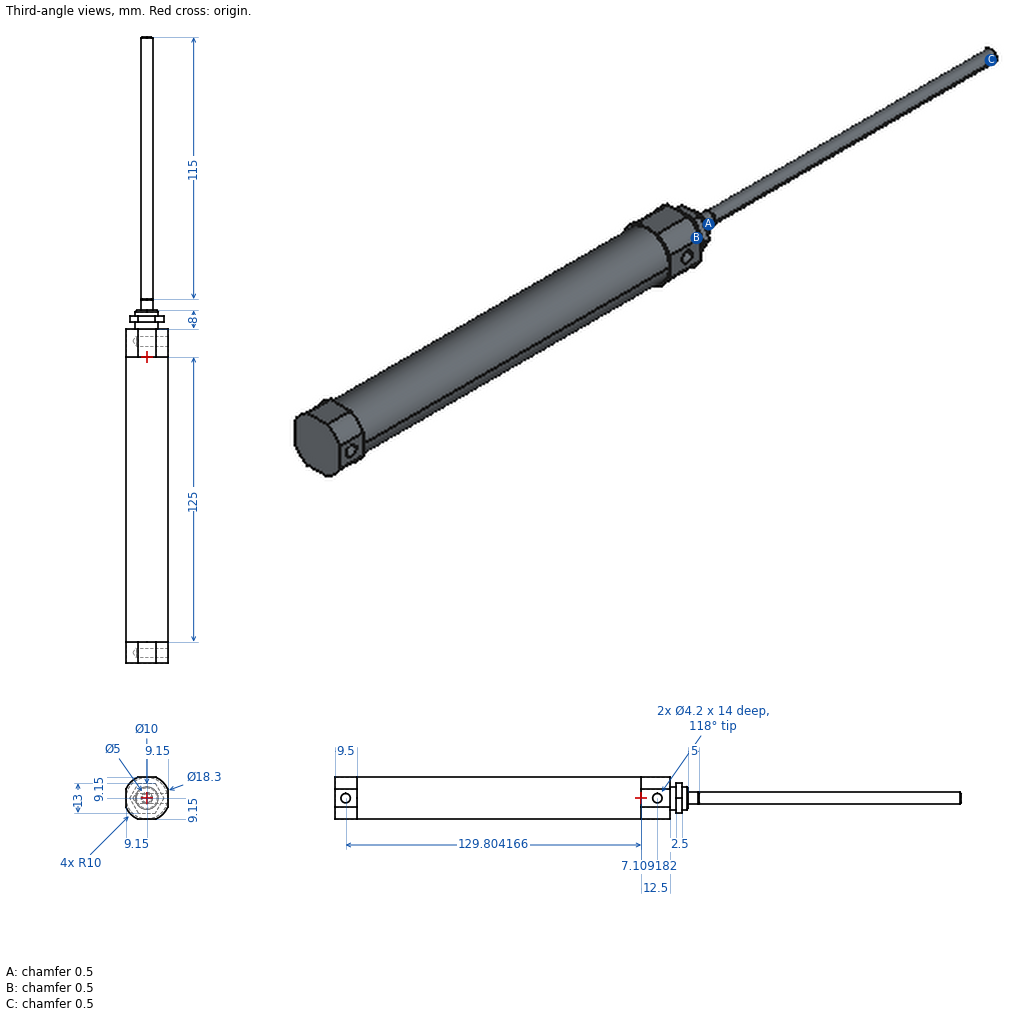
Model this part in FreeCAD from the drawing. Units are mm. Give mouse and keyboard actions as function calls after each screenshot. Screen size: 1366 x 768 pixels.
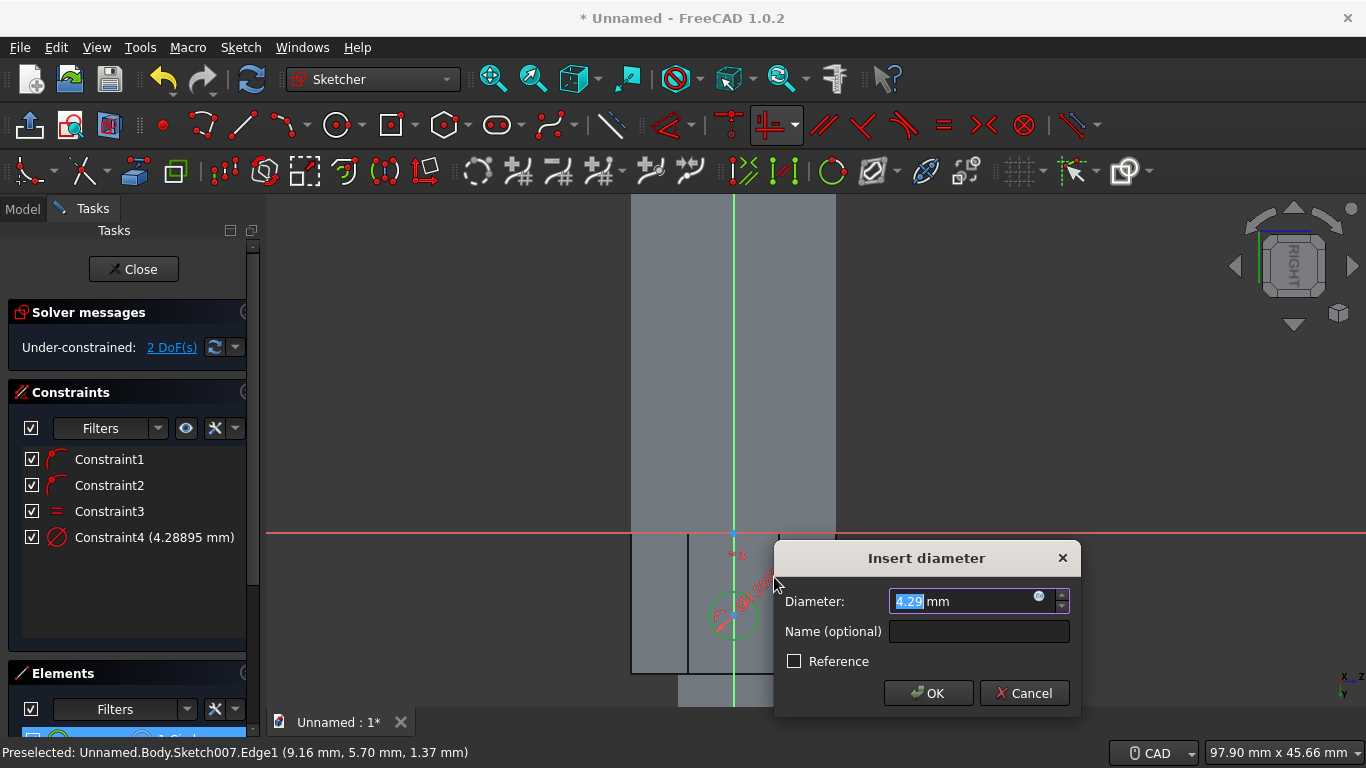
text(4.2)
key(Return)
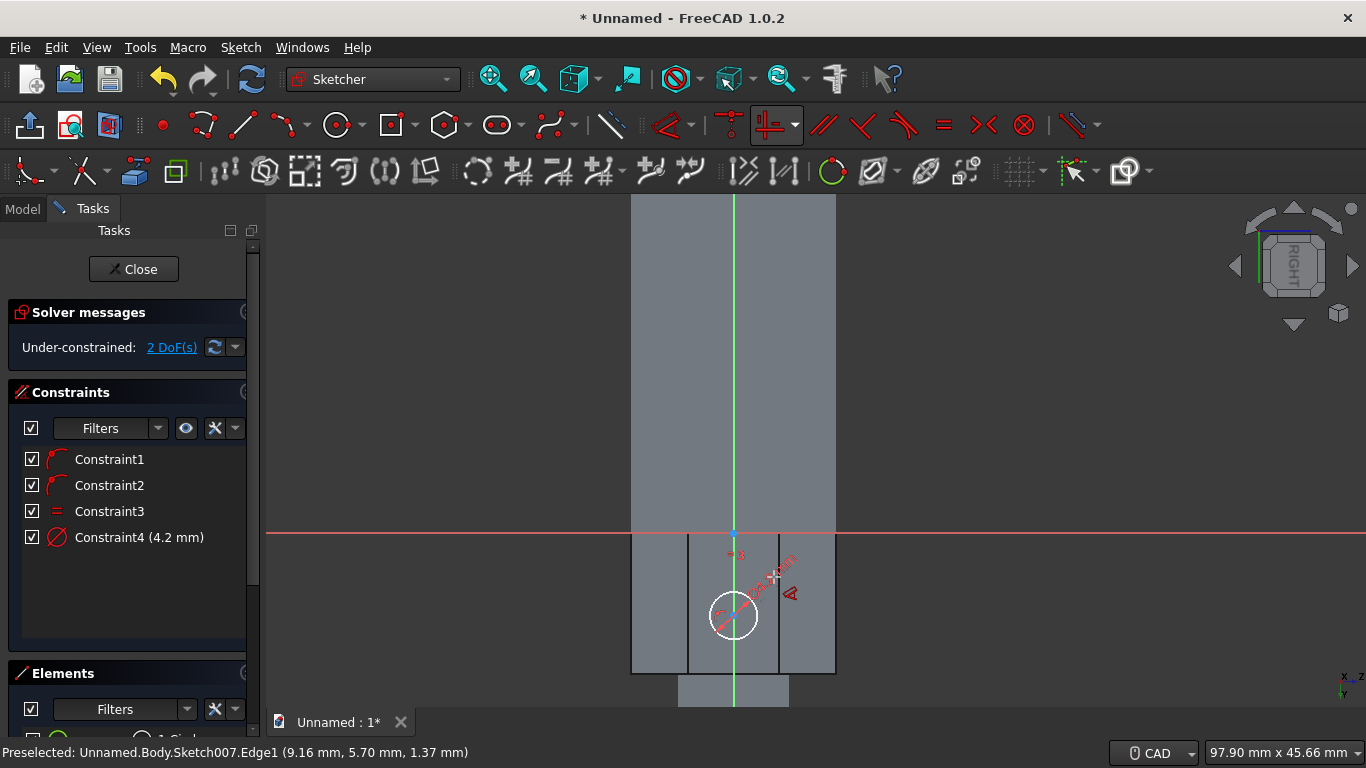
click(734, 616)
click(768, 555)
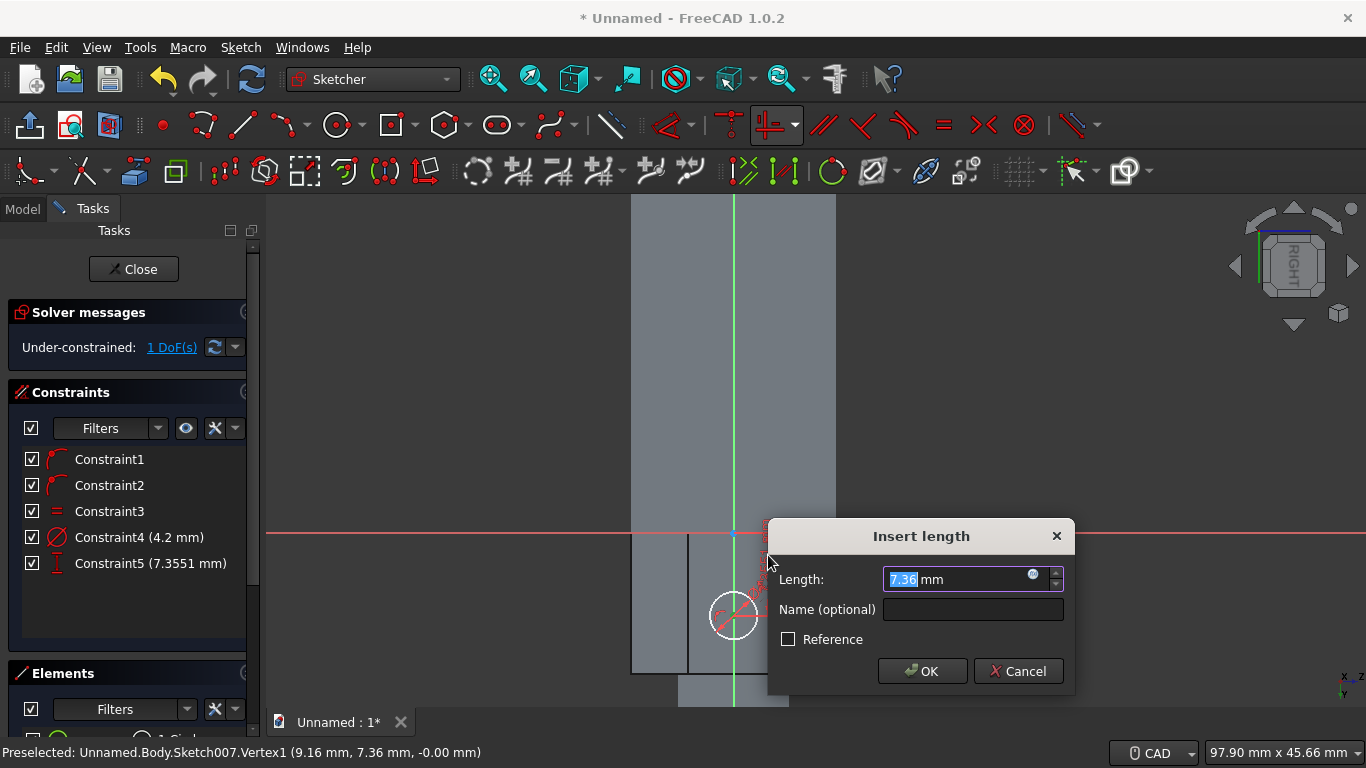
text(7.109182)
key(Return)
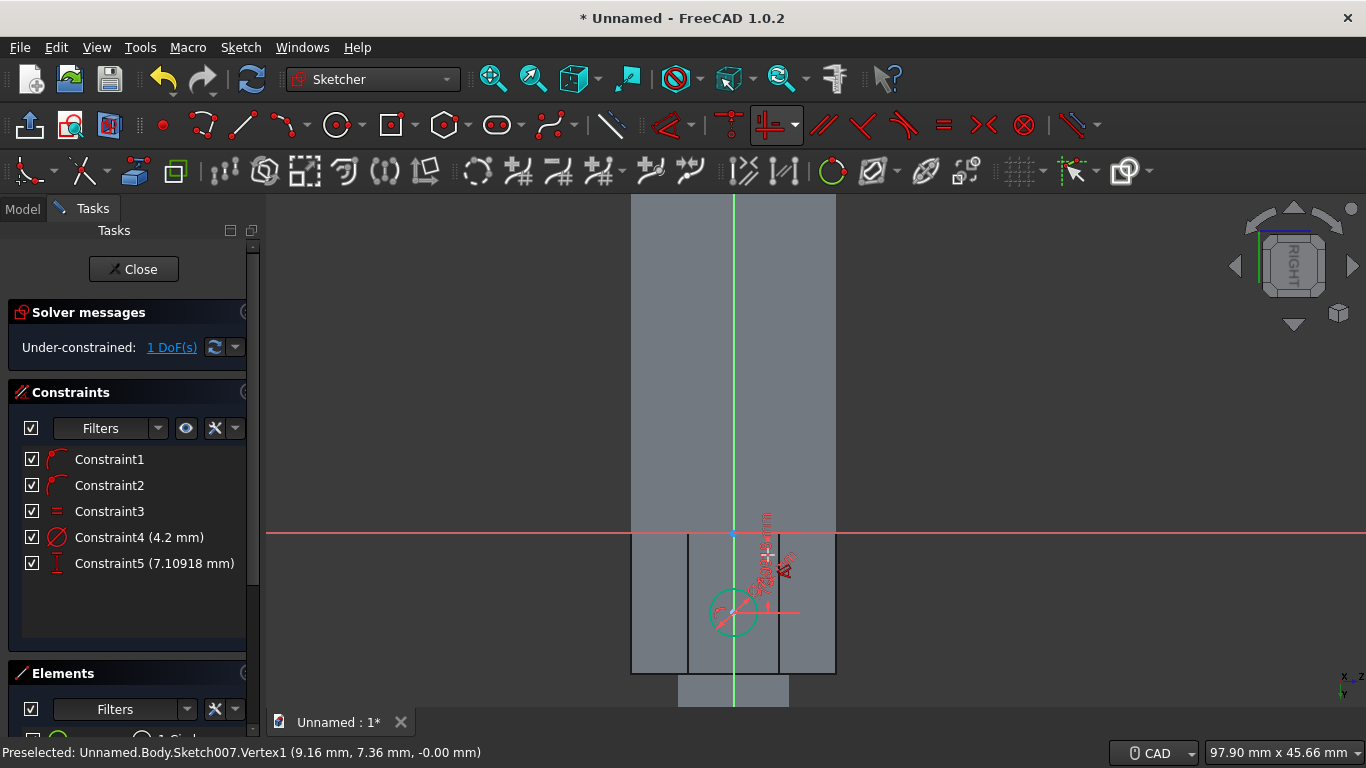
scroll(751, 604, down, 8)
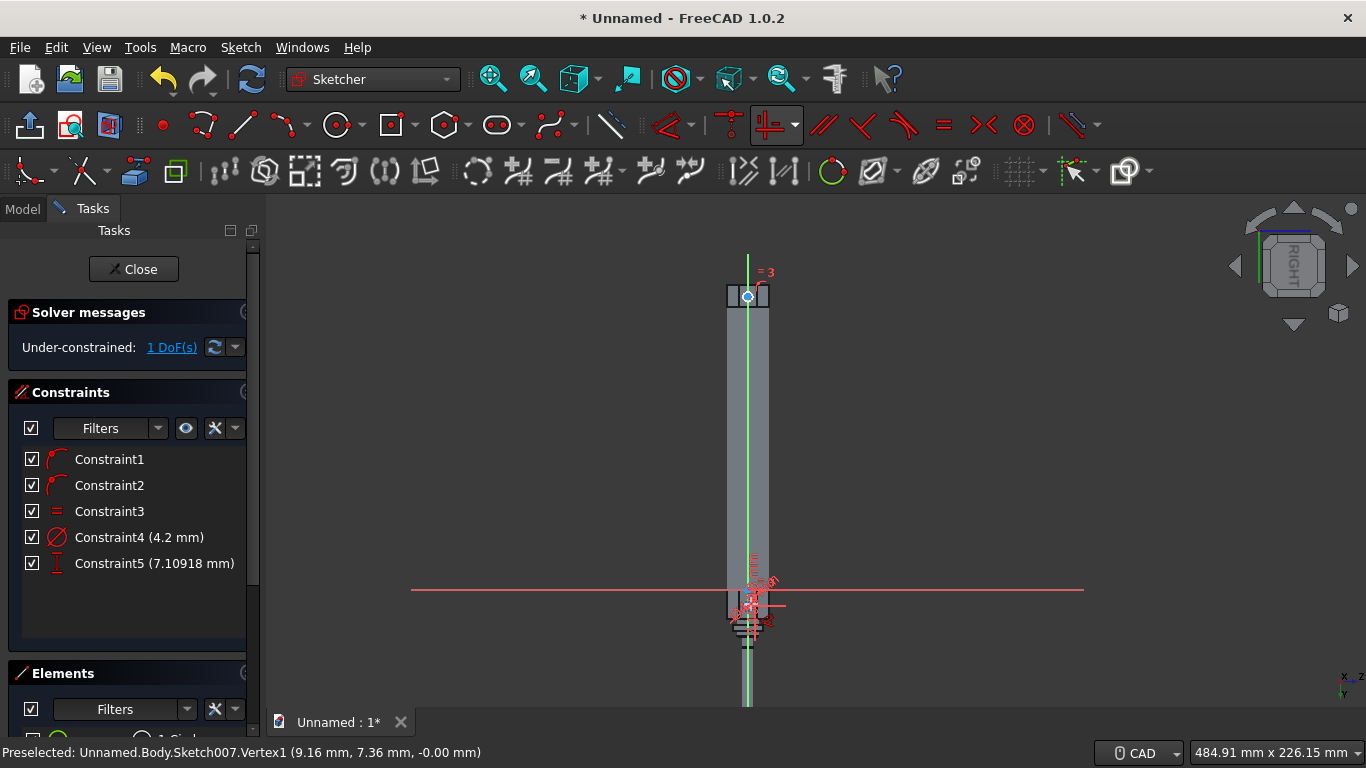
click(748, 297)
click(782, 444)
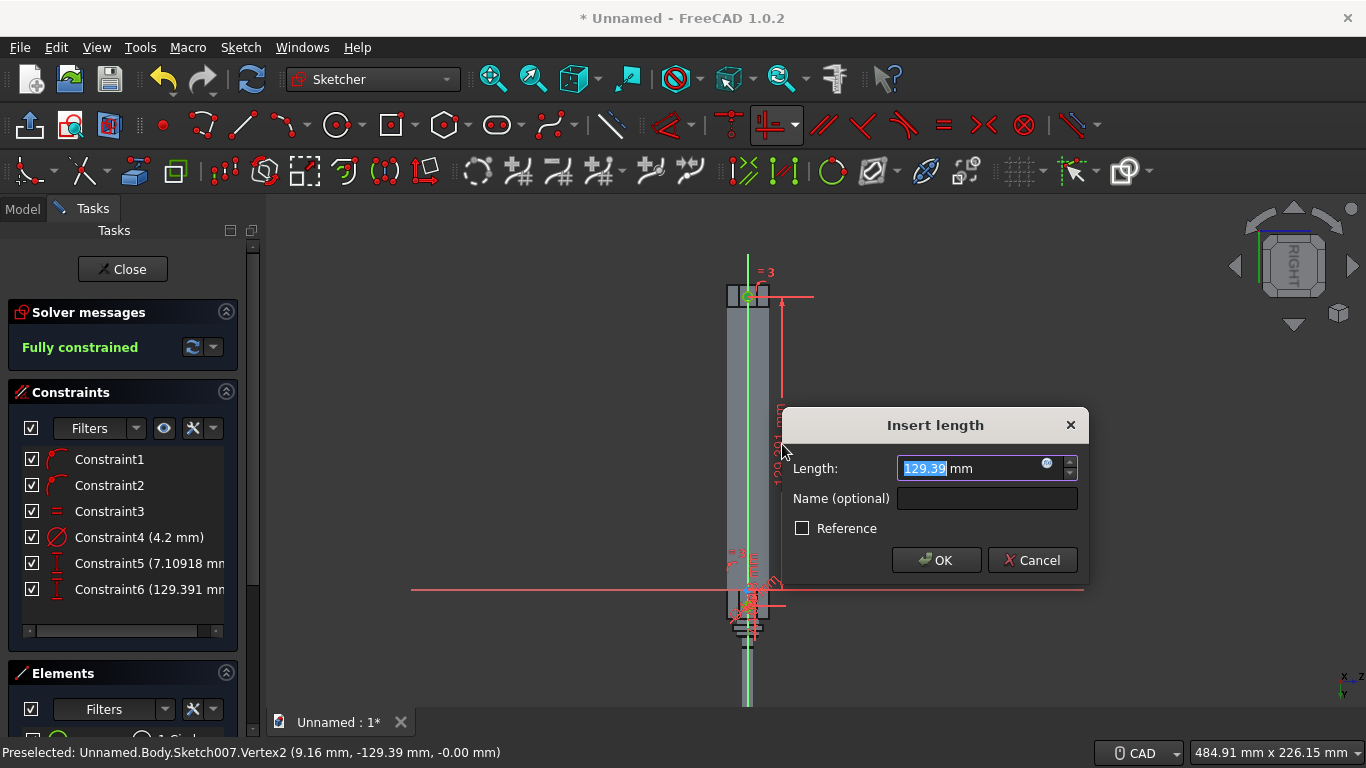
text(129.804166)
key(Return)
key(Escape)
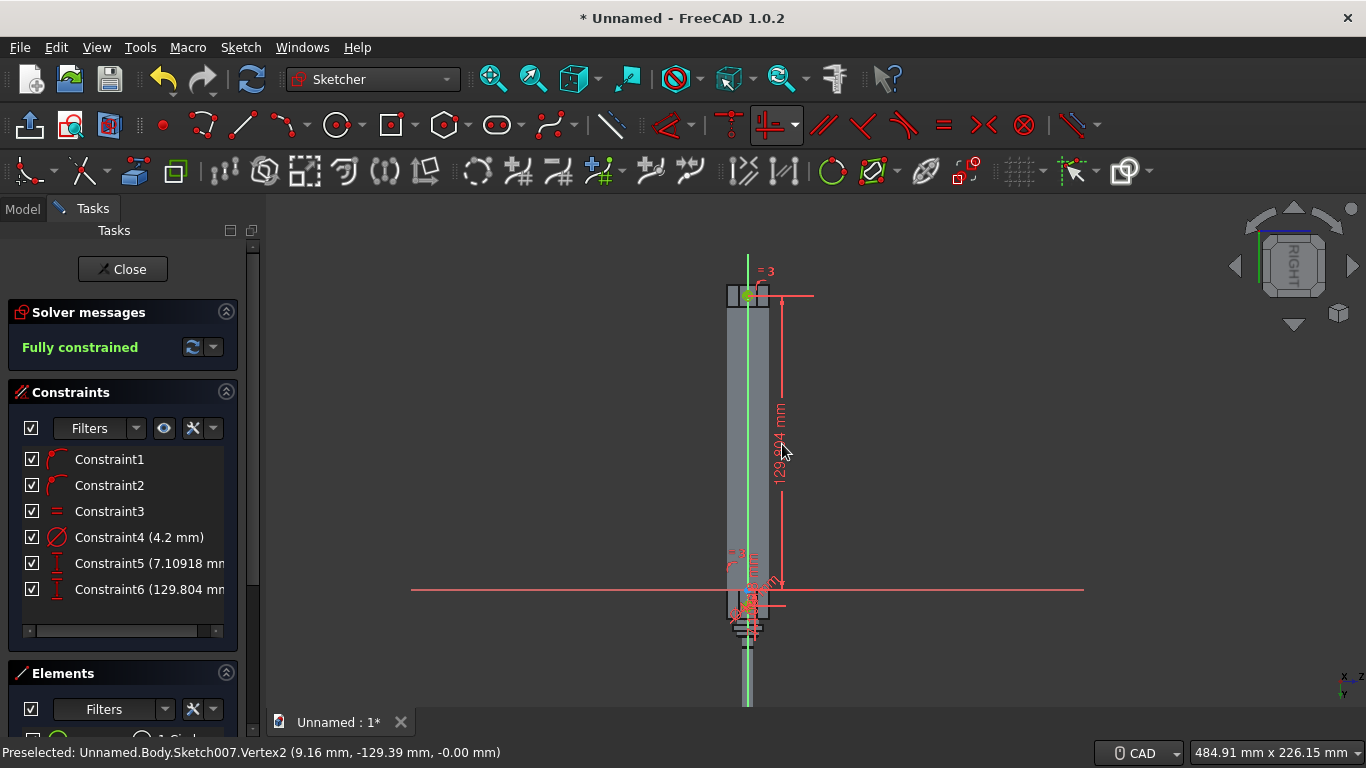
click(123, 269)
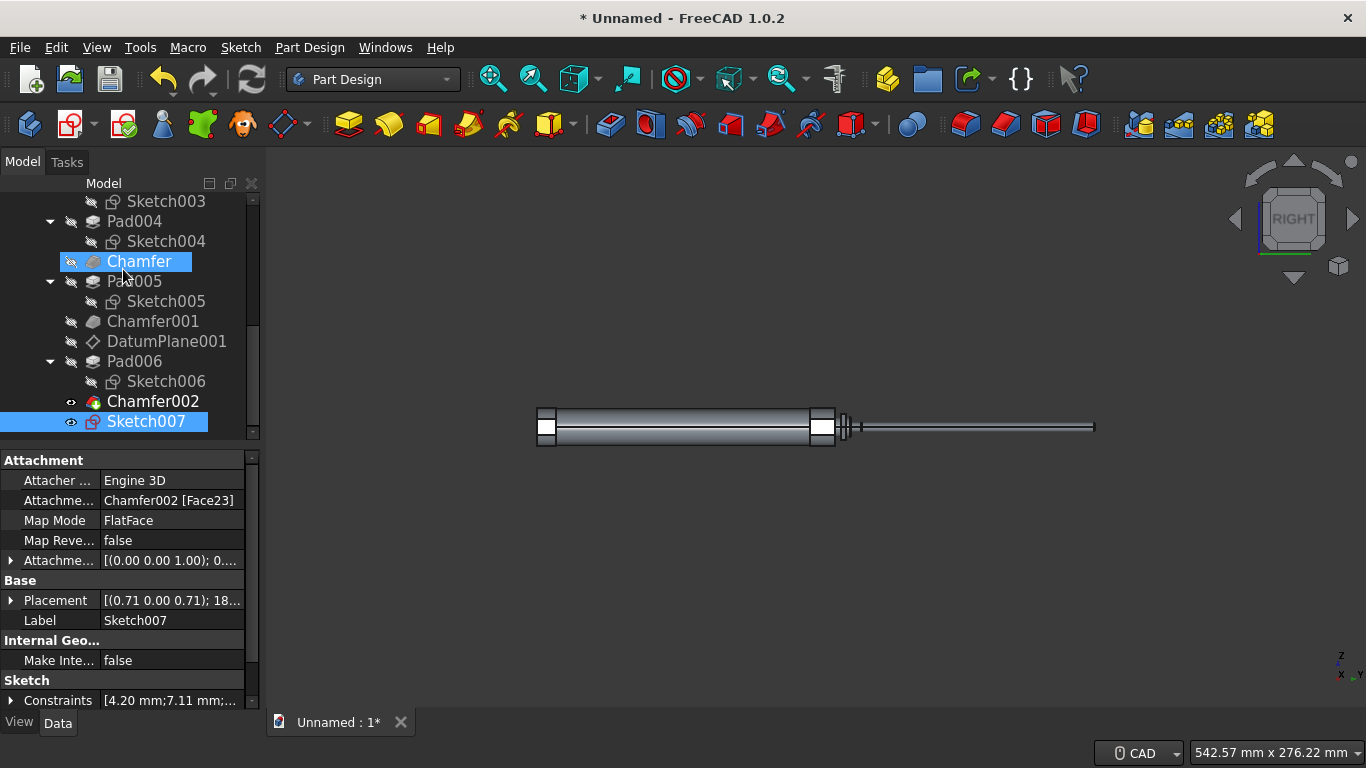
click(652, 124)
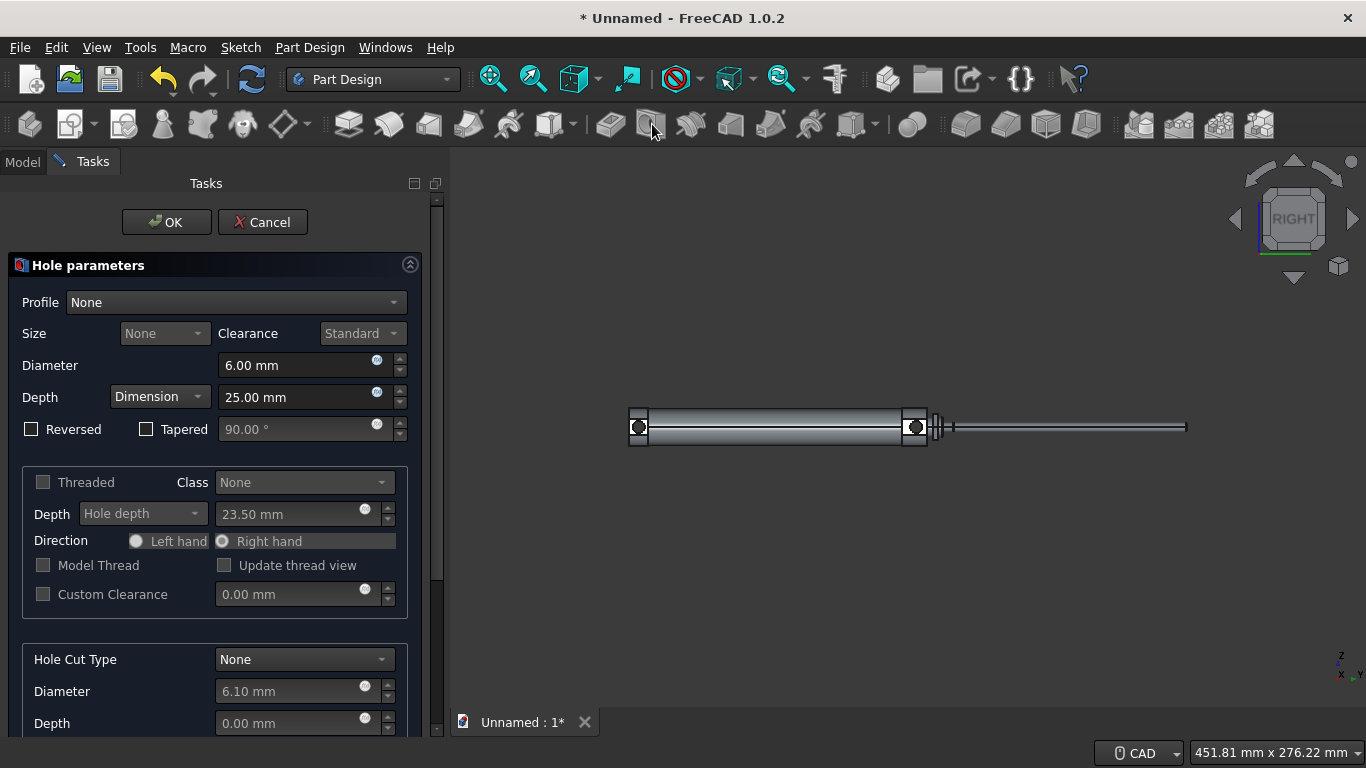
triple_click(305, 365)